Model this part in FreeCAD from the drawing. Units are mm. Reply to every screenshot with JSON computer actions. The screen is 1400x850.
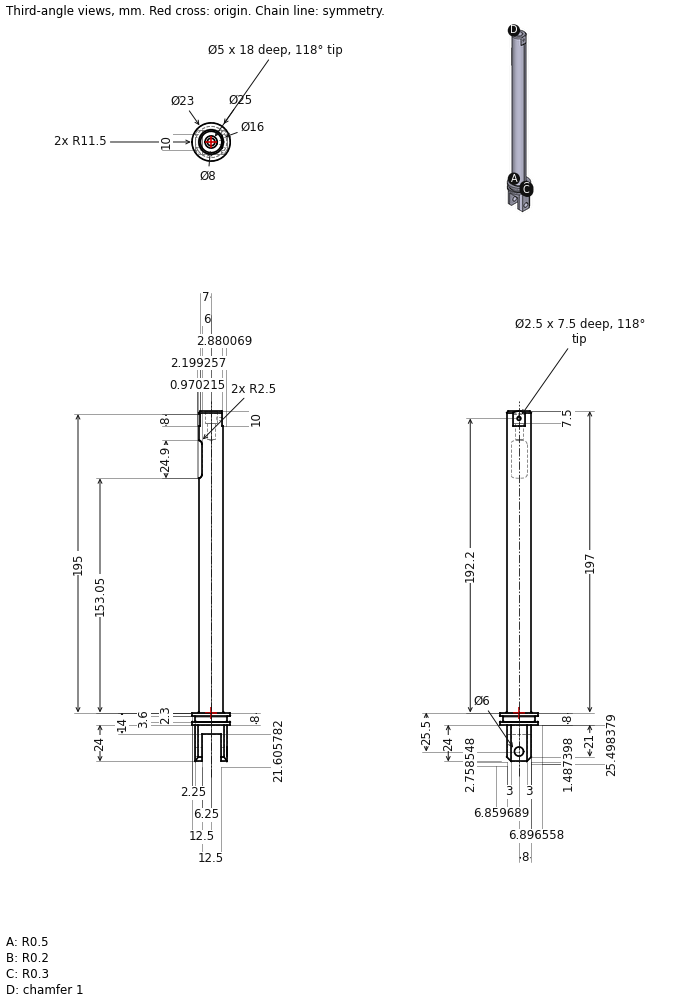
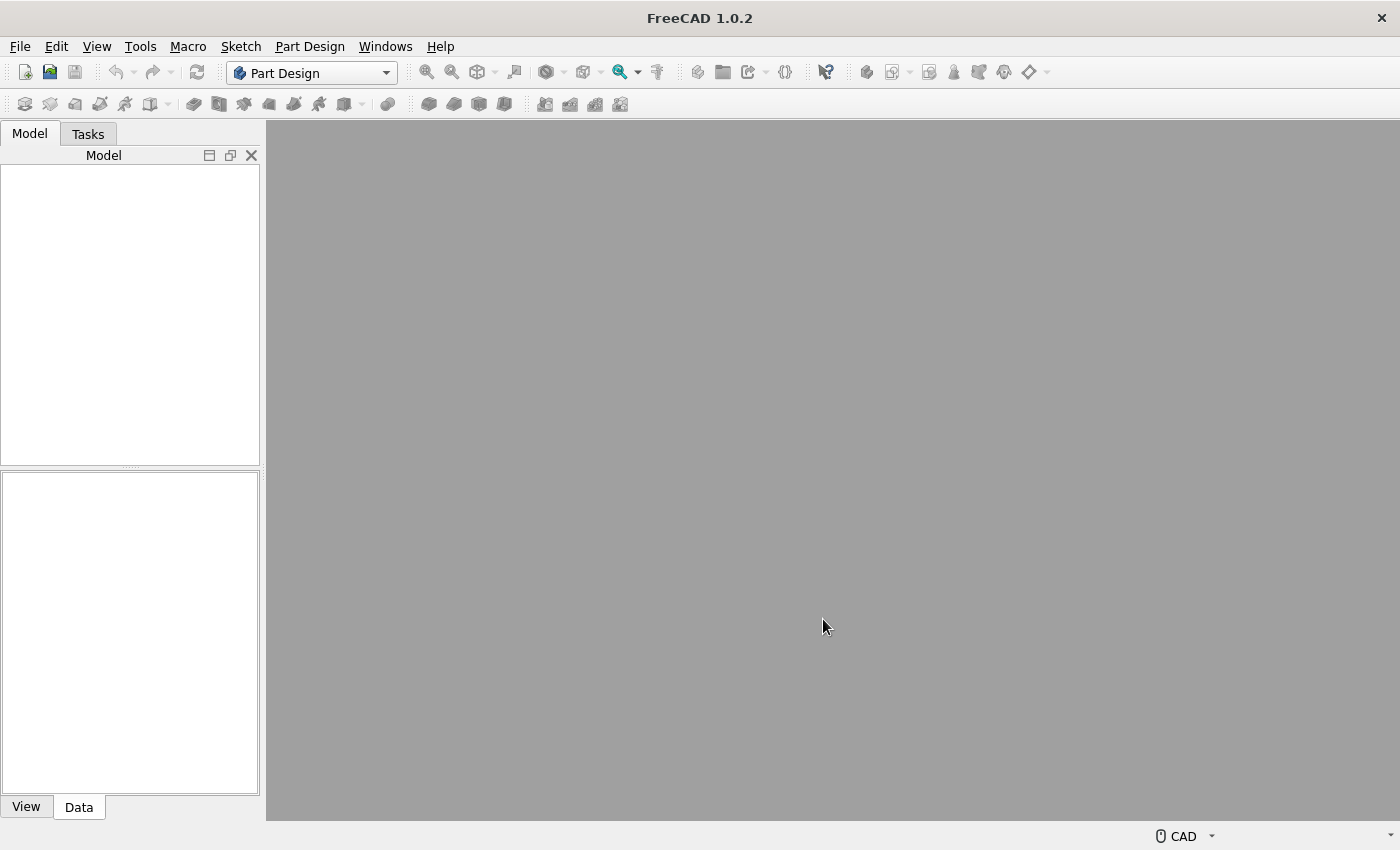
{"action": "left_click", "coordinate": [25, 72]}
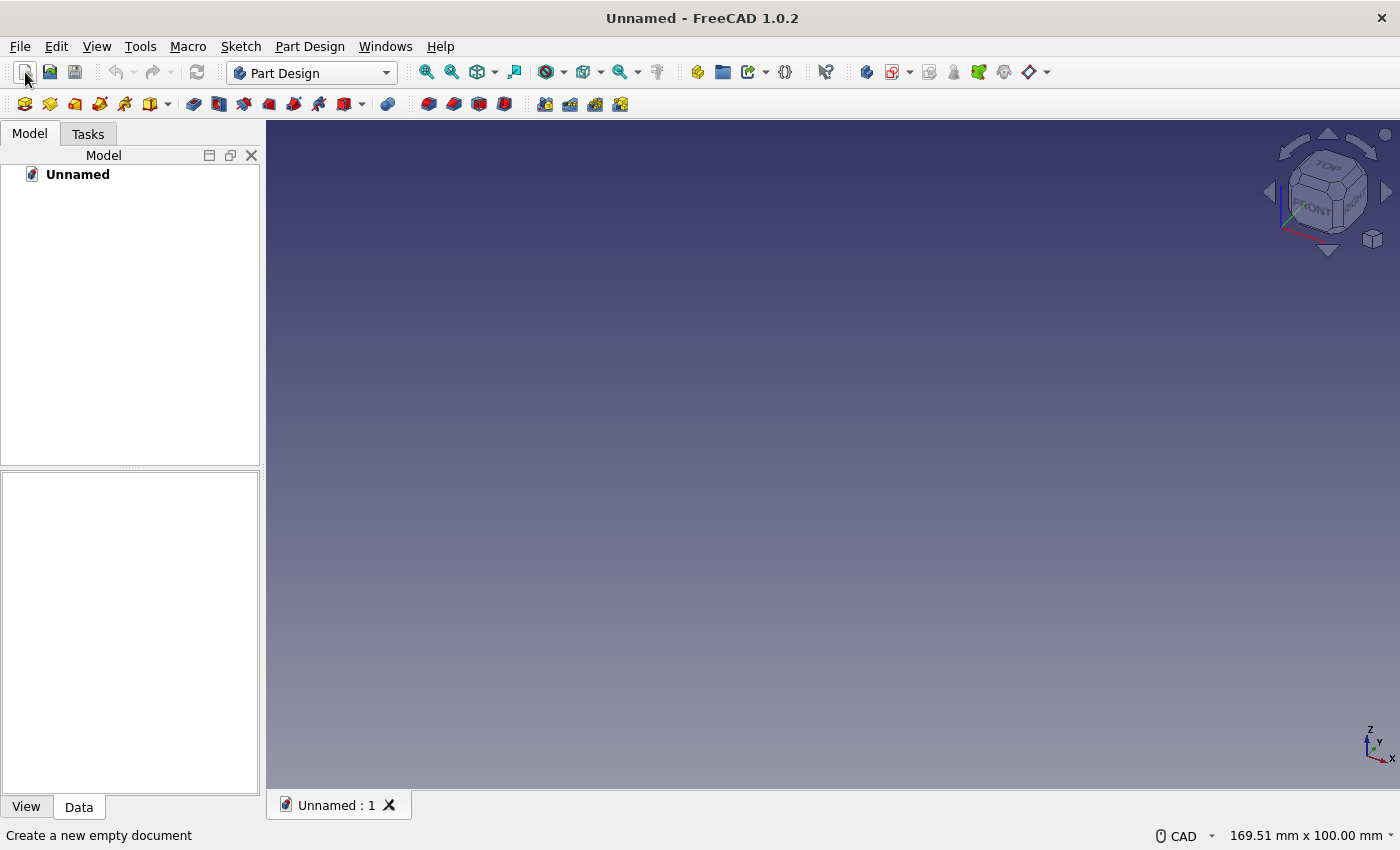
{"action": "left_click", "coordinate": [892, 72]}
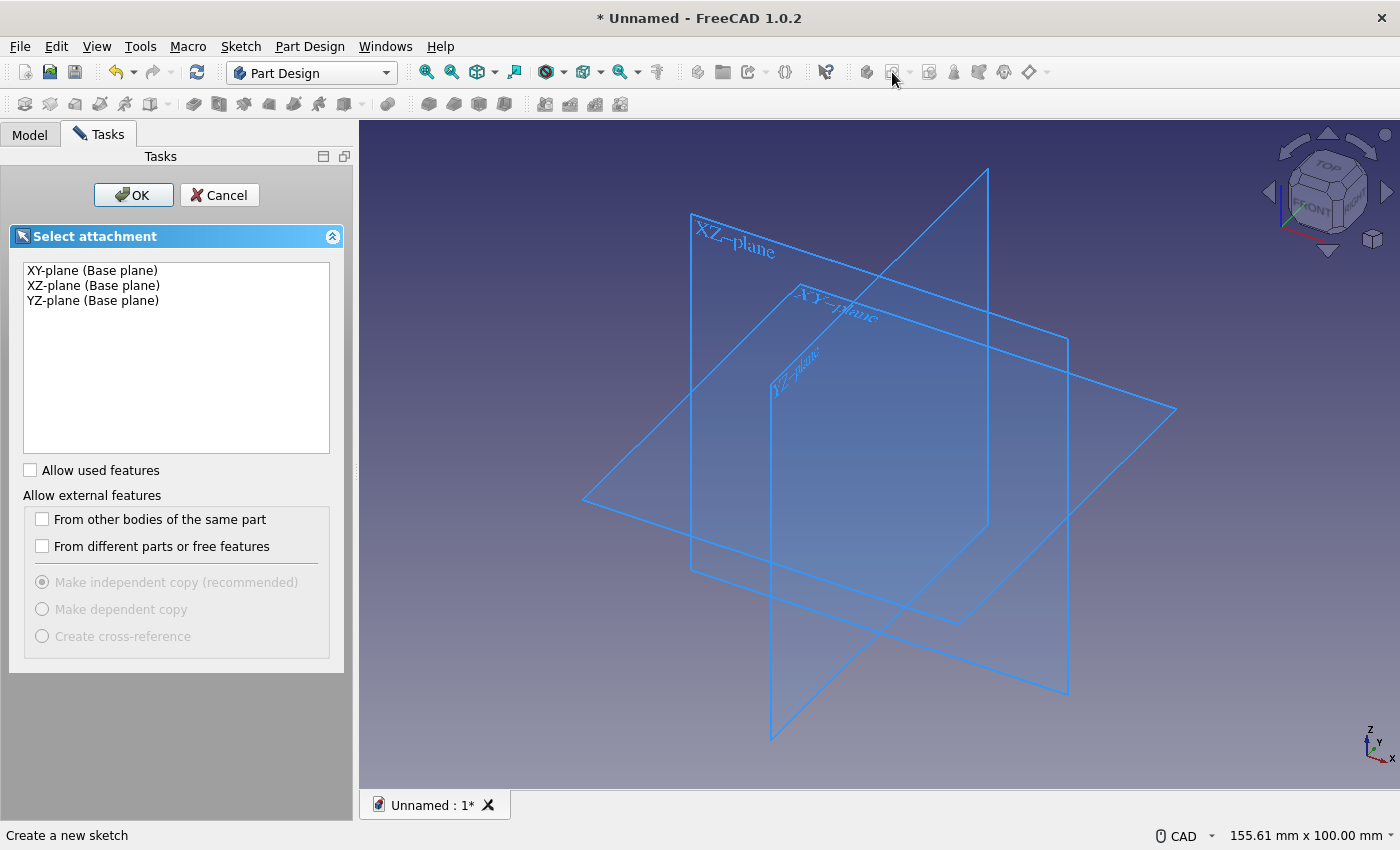
{"action": "left_click", "coordinate": [84, 270]}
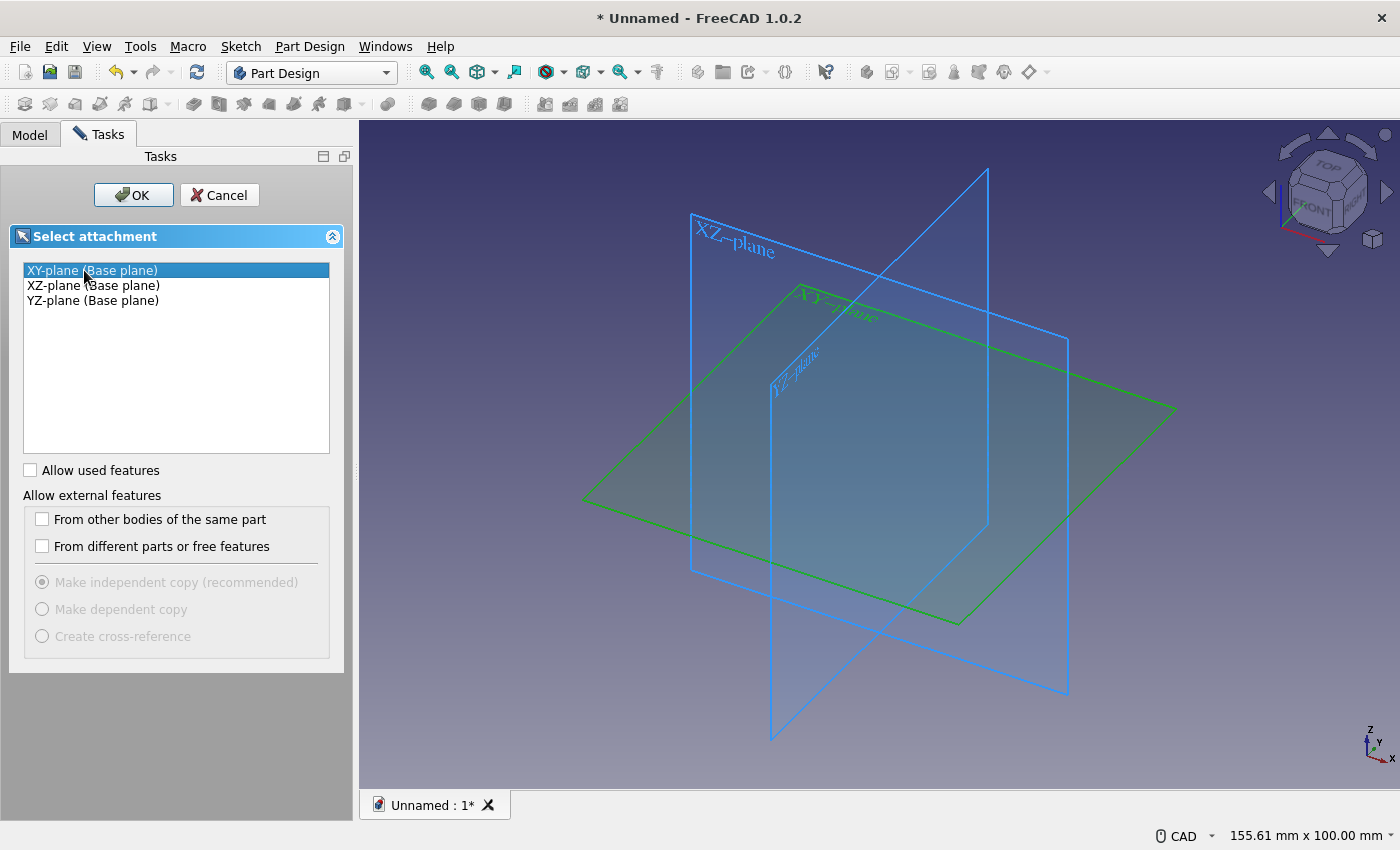
{"action": "left_click", "coordinate": [134, 195]}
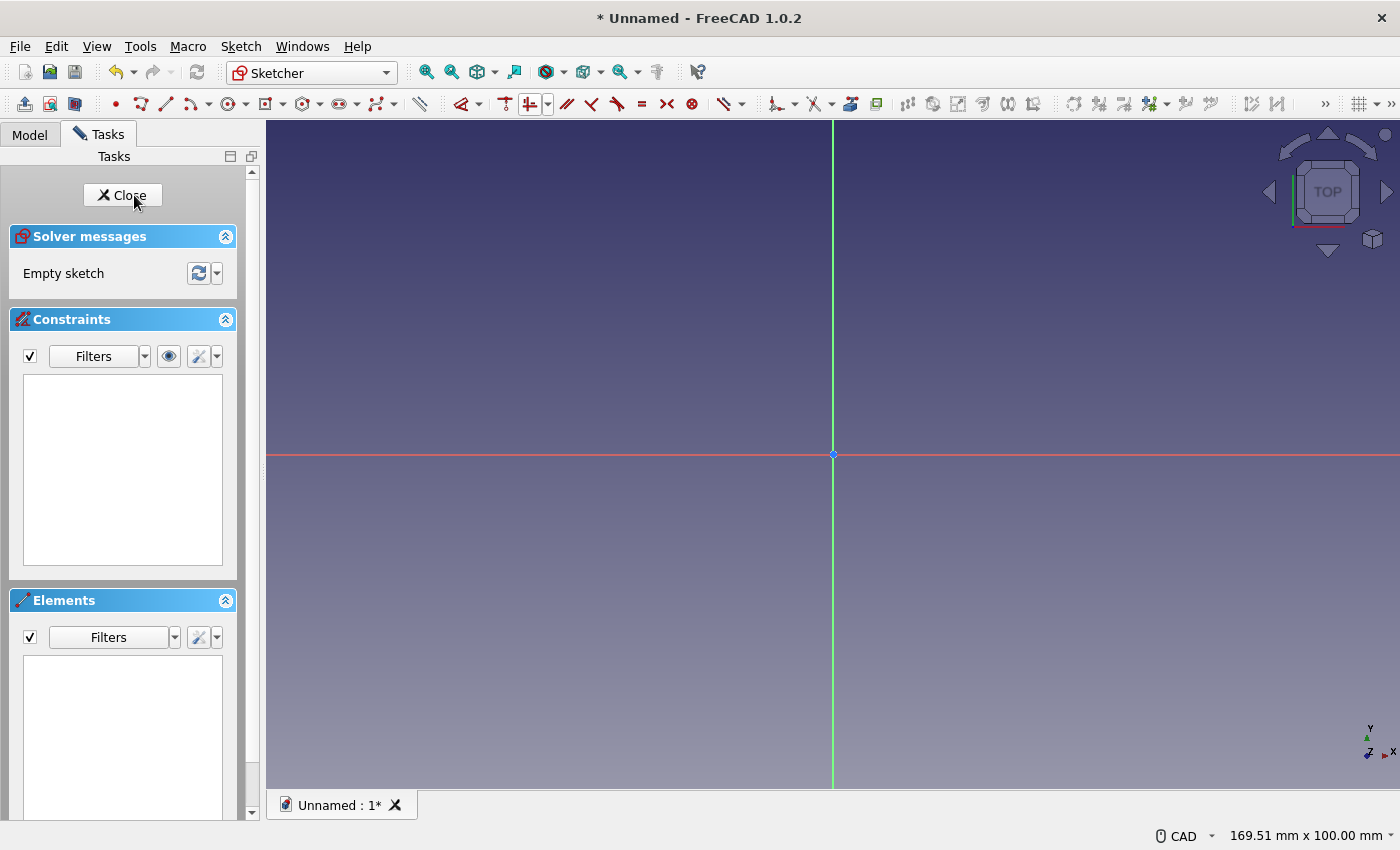
{"action": "scroll", "coordinate": [855, 454], "scroll_direction": "up", "scroll_amount": 7}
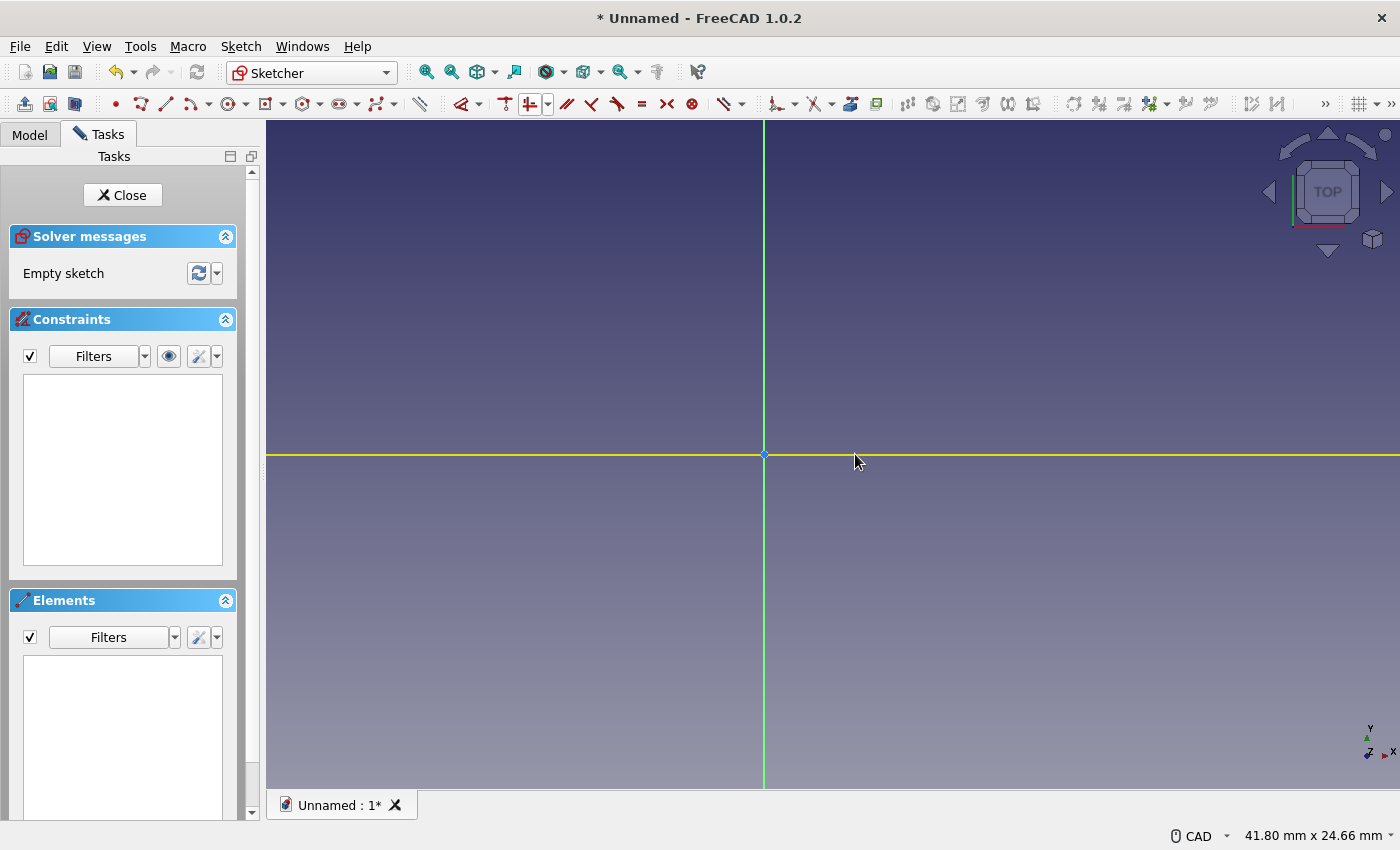
{"action": "left_click", "coordinate": [228, 104]}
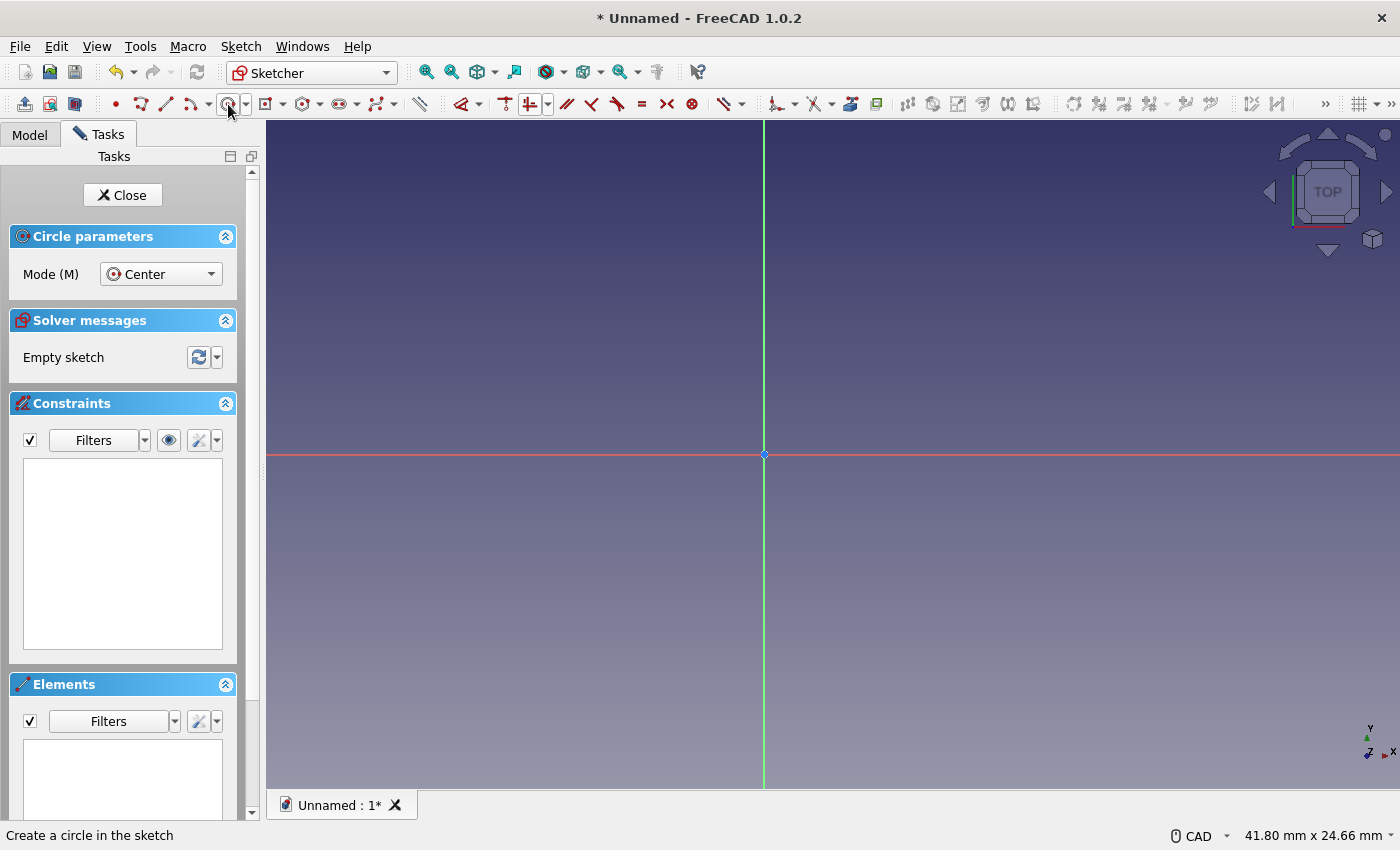
{"action": "left_click", "coordinate": [764, 454]}
{"action": "mouse_move", "coordinate": [918, 301]}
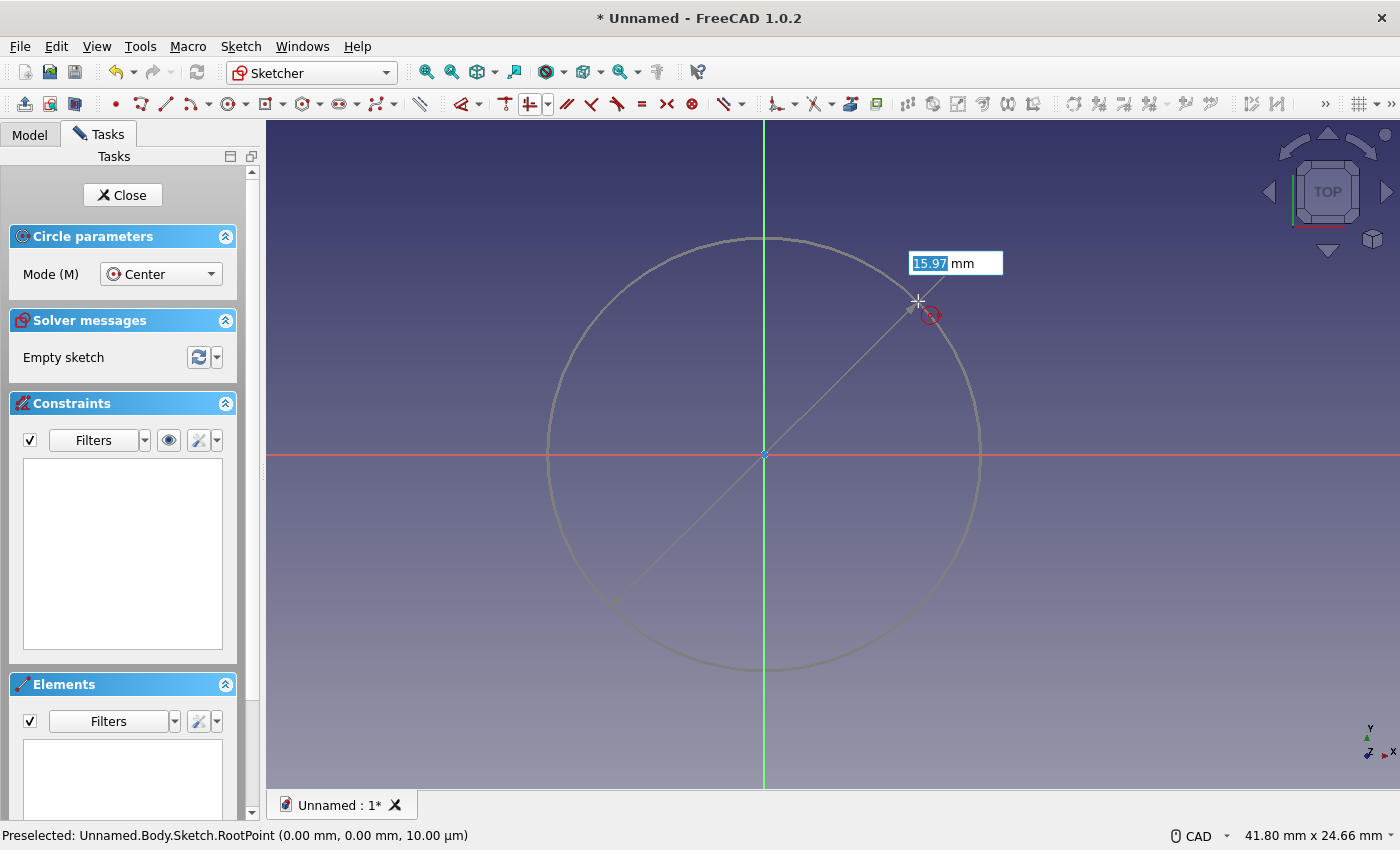
{"action": "type", "text": "16"}
{"action": "key", "text": "Return"}
{"action": "key", "text": "Escape"}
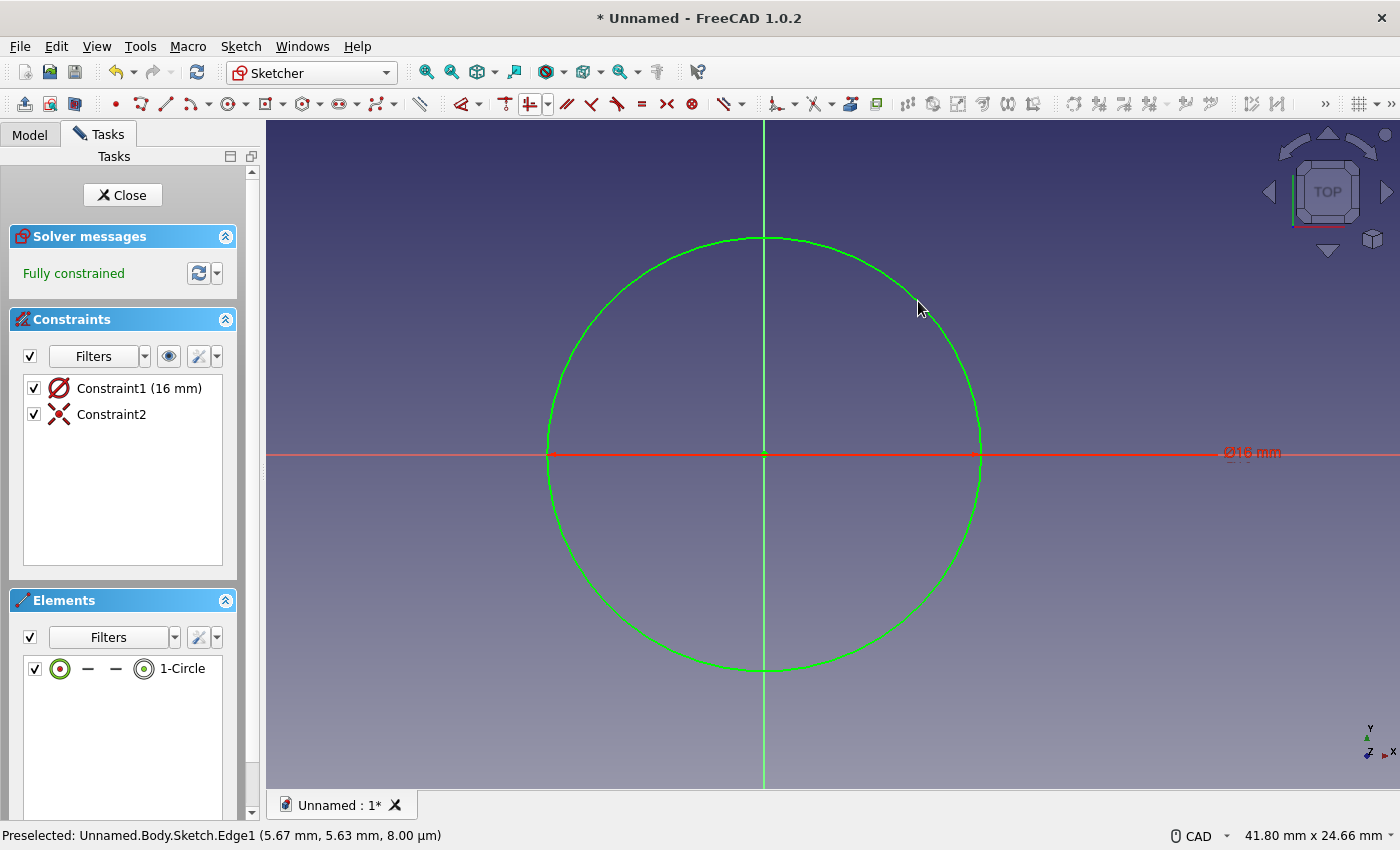
{"action": "left_click", "coordinate": [123, 195]}